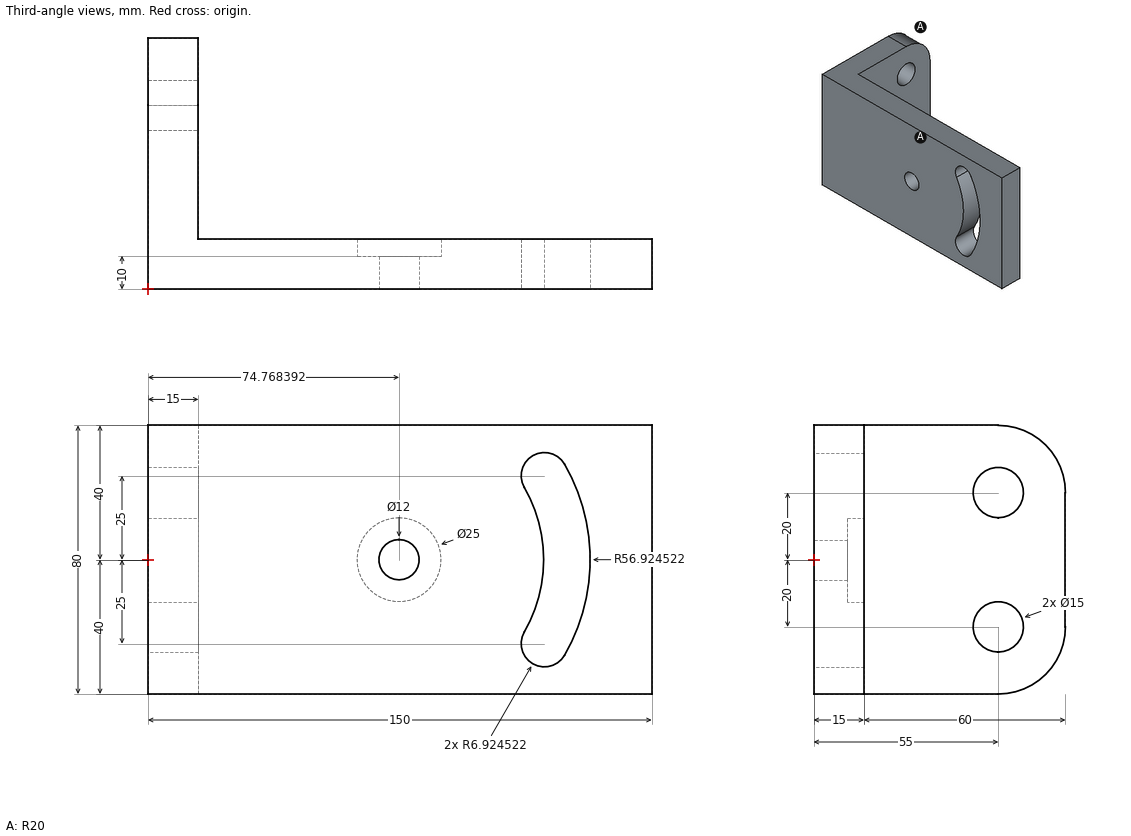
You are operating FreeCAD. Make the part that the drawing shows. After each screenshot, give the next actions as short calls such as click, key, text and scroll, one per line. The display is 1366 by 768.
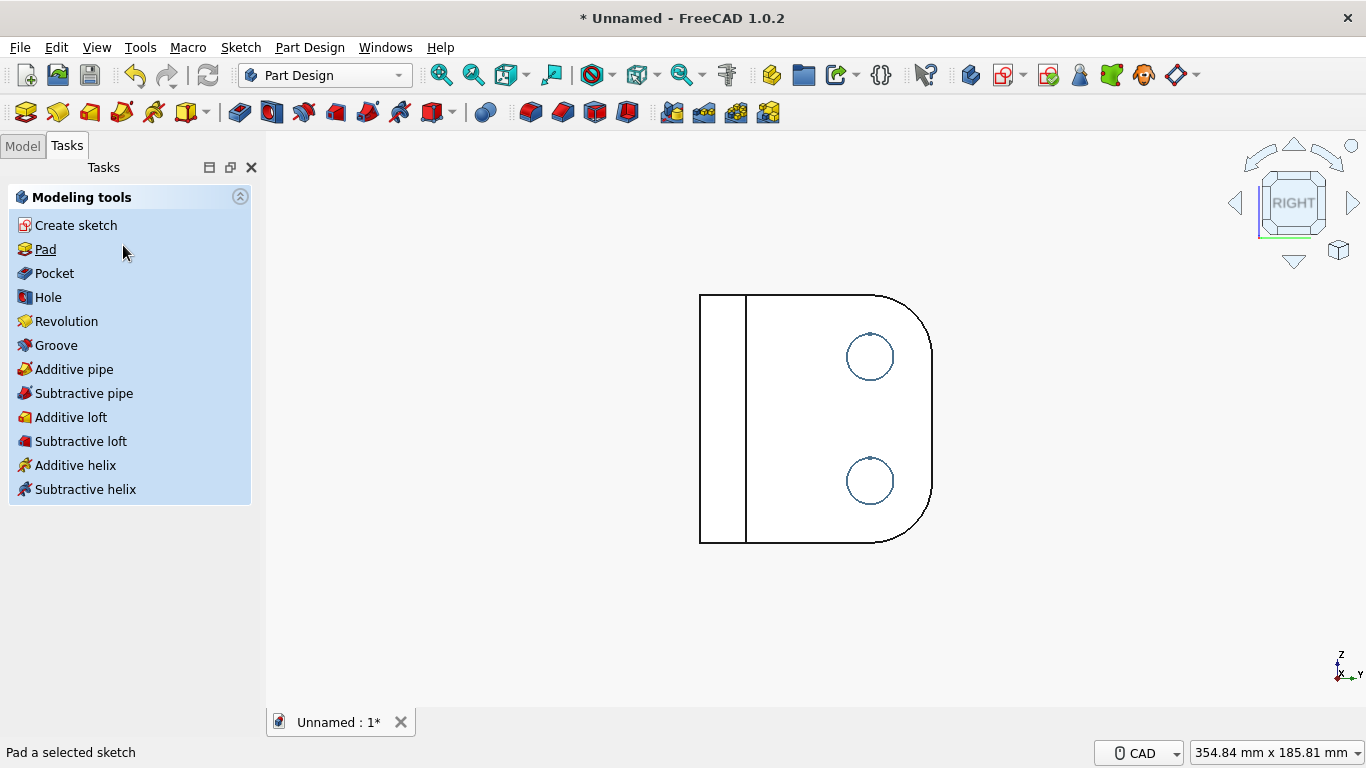
click(240, 112)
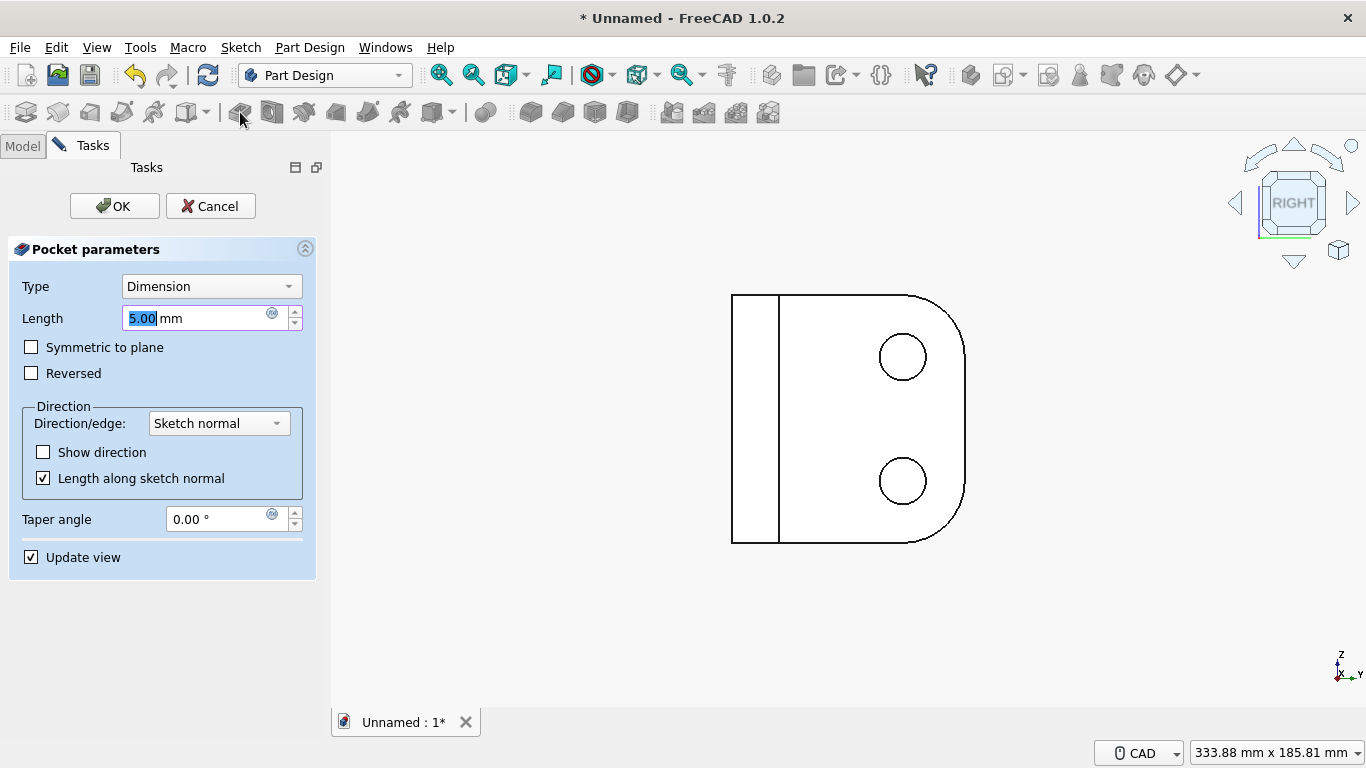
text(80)
key(Tab)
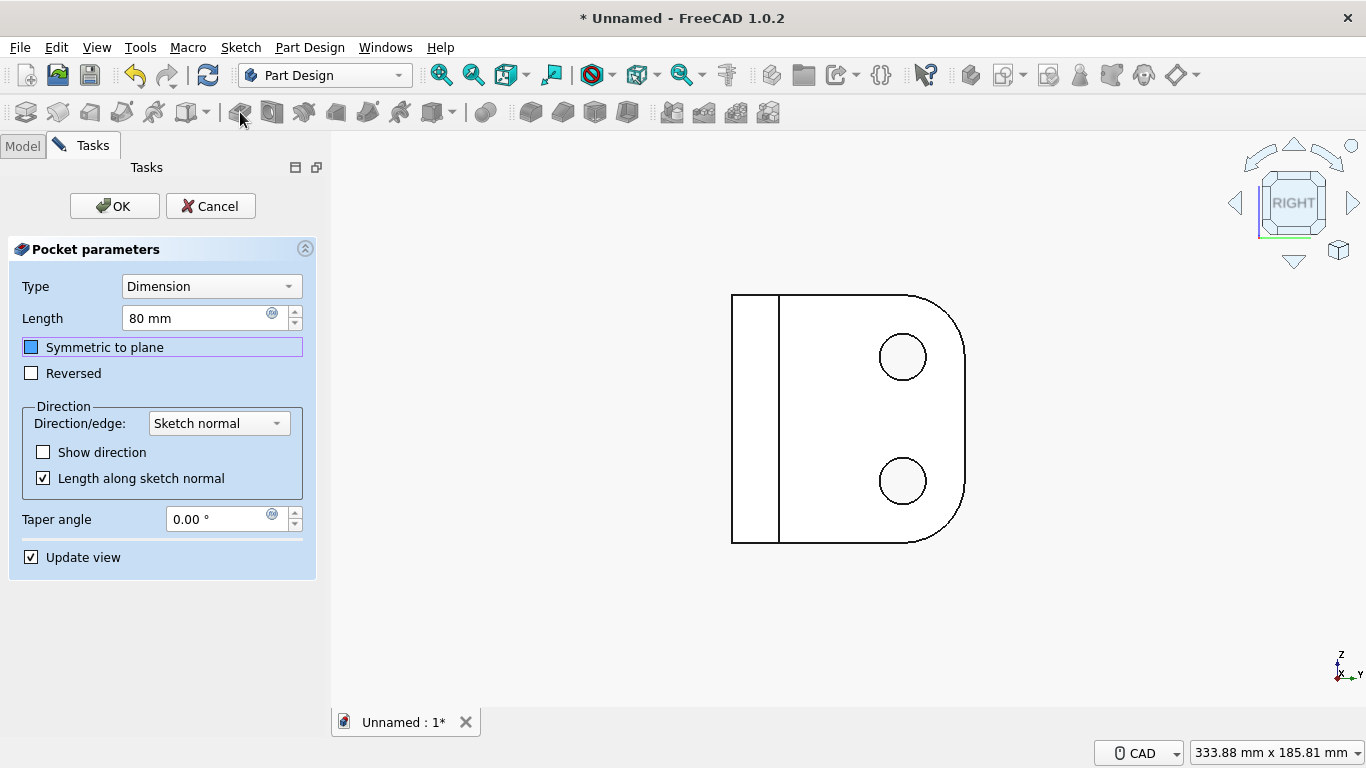
click(30, 347)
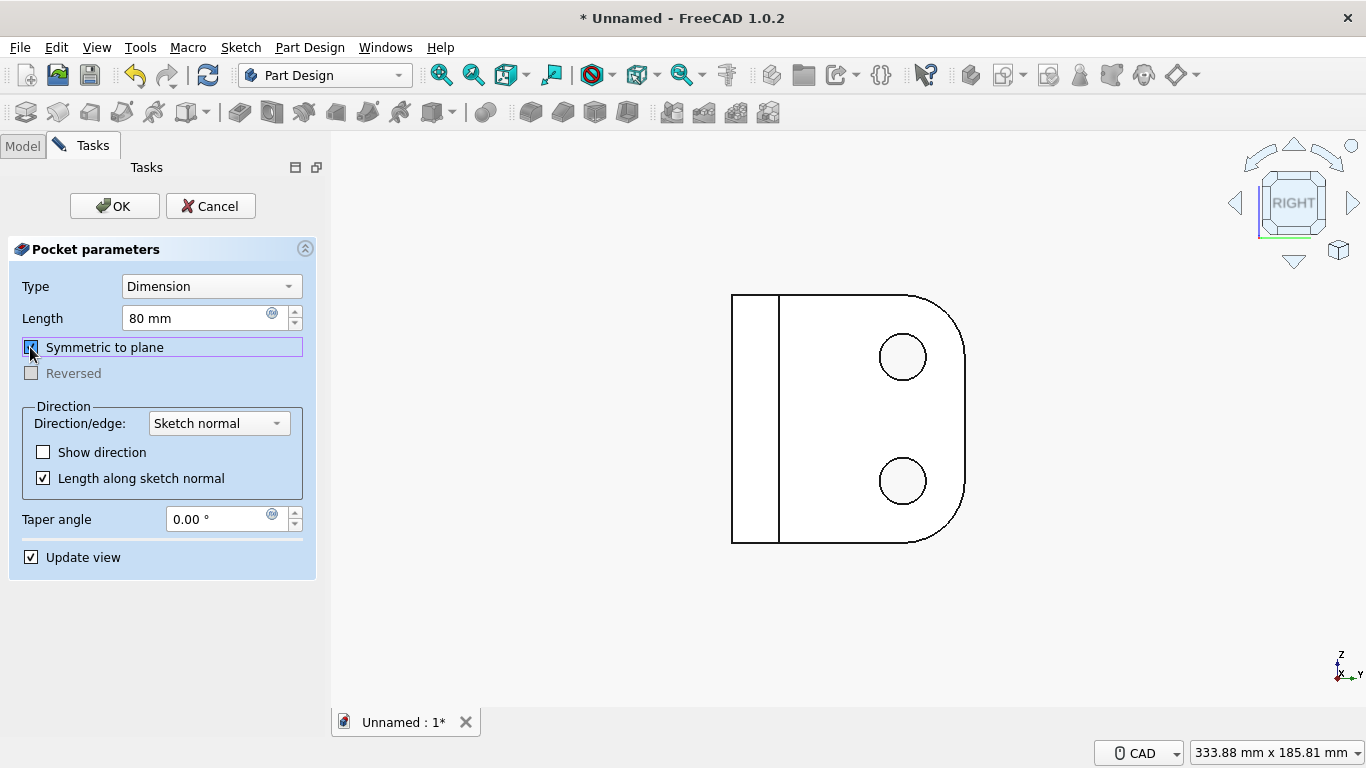
click(115, 206)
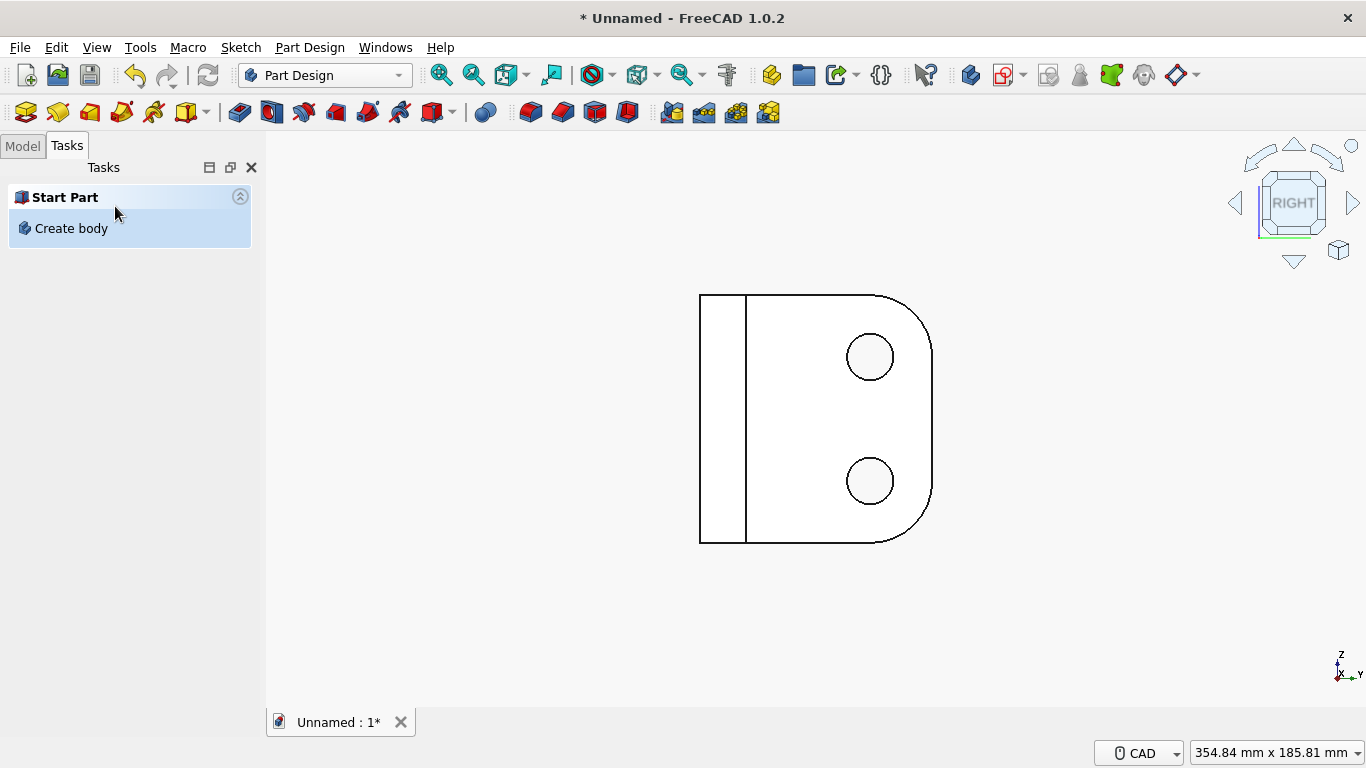
key(0)